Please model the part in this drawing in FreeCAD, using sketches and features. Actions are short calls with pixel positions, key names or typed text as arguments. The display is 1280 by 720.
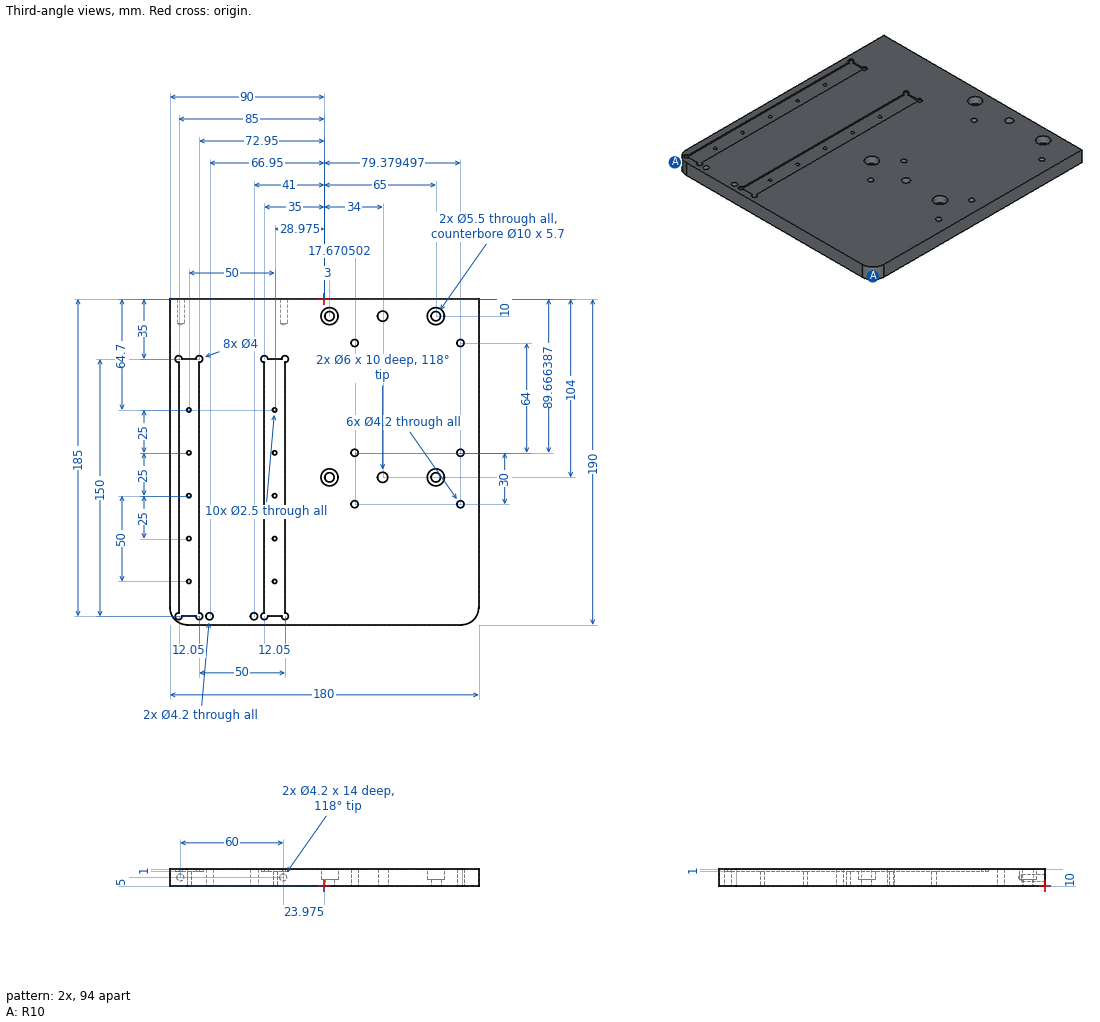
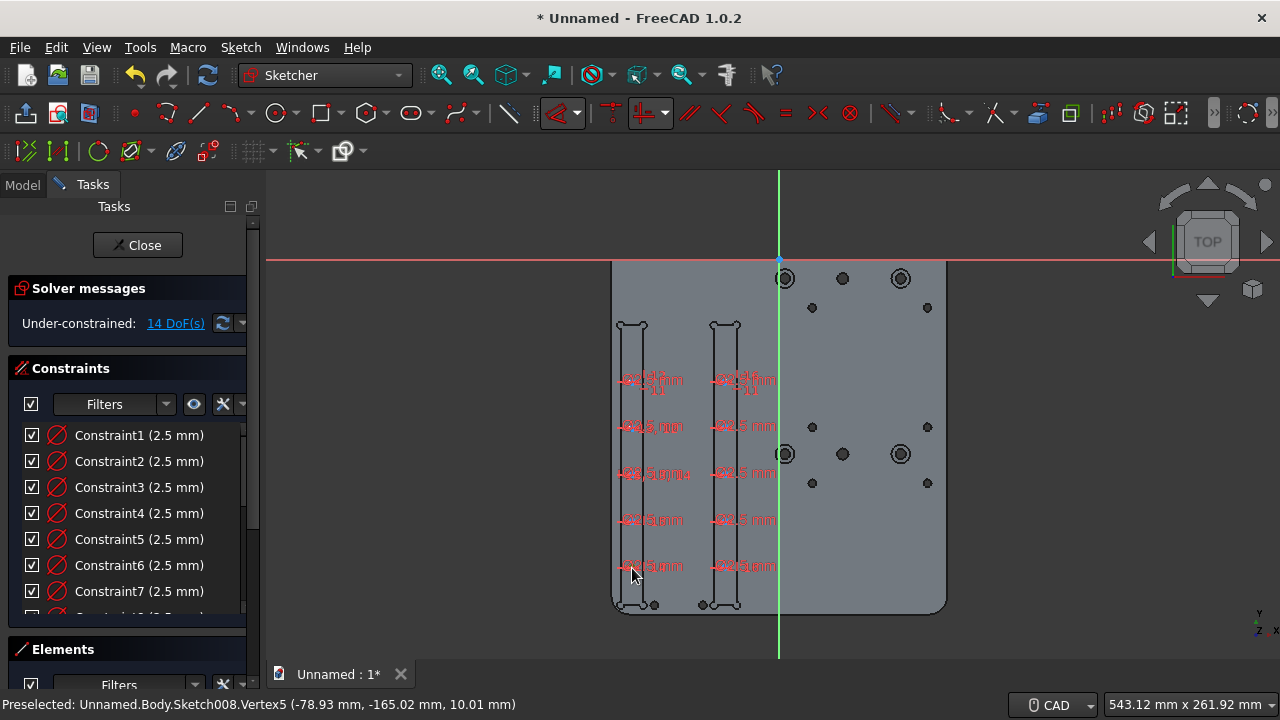
click(725, 568)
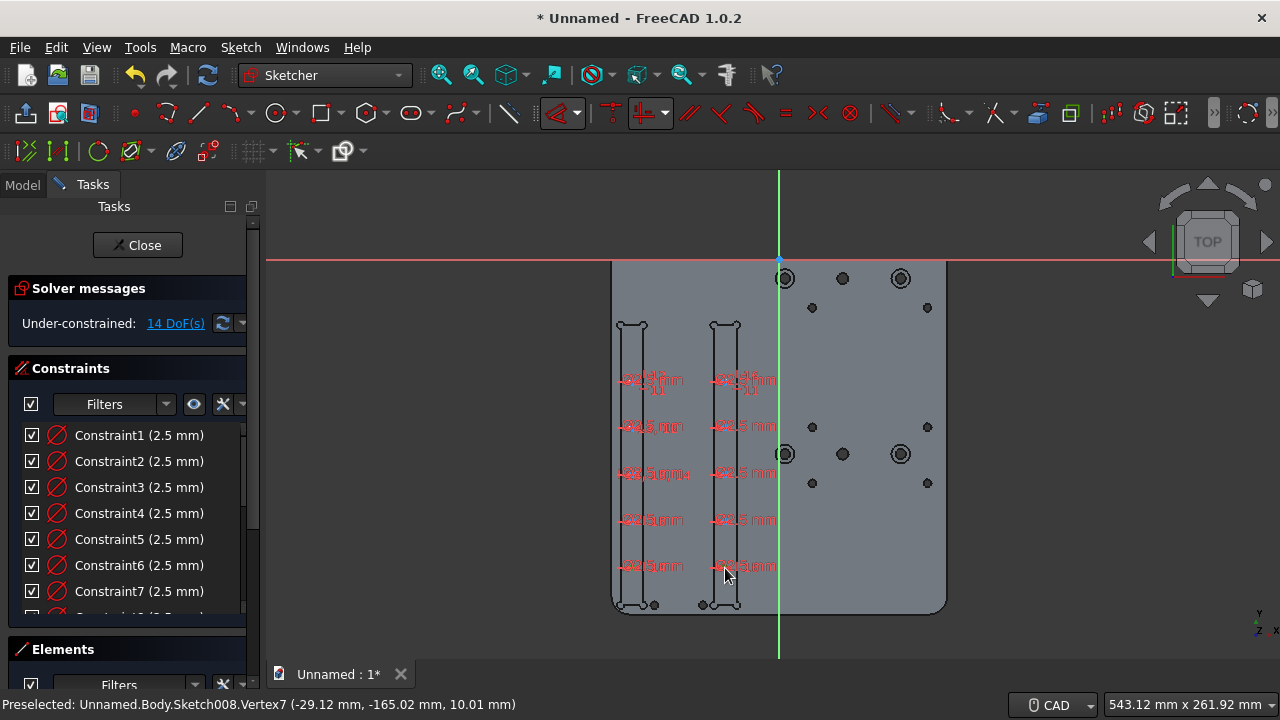
key(h)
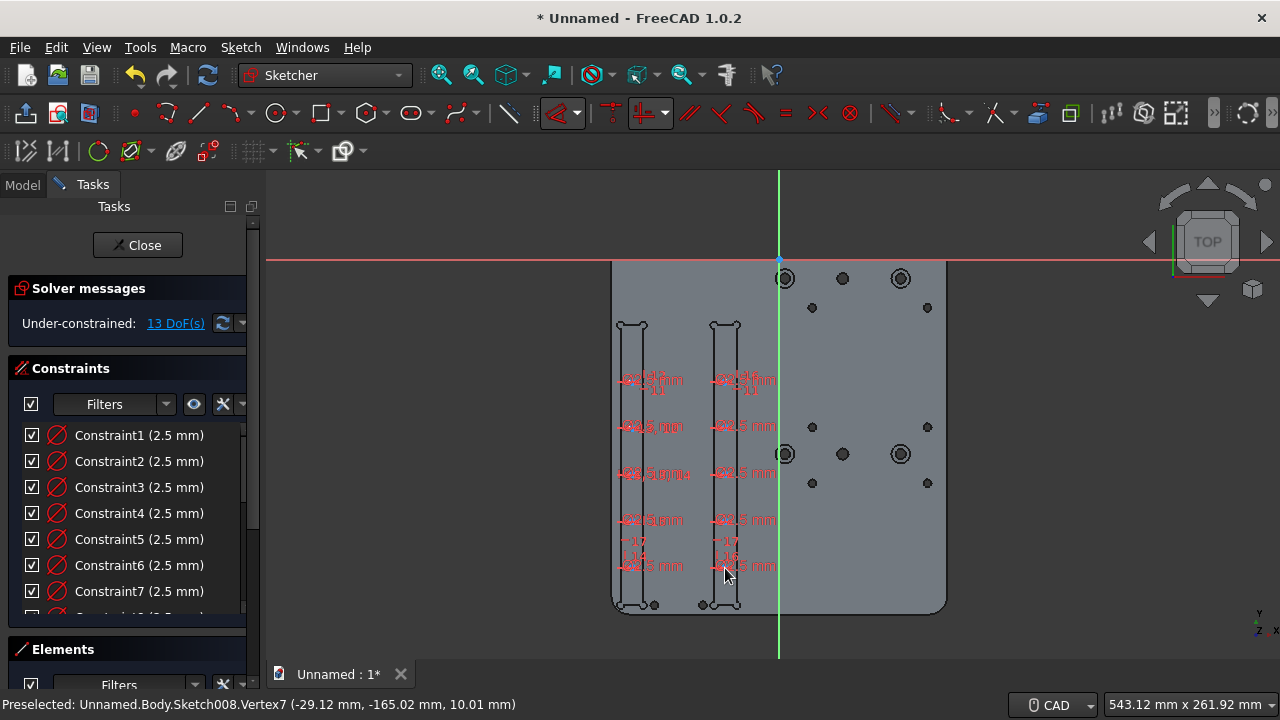
click(725, 568)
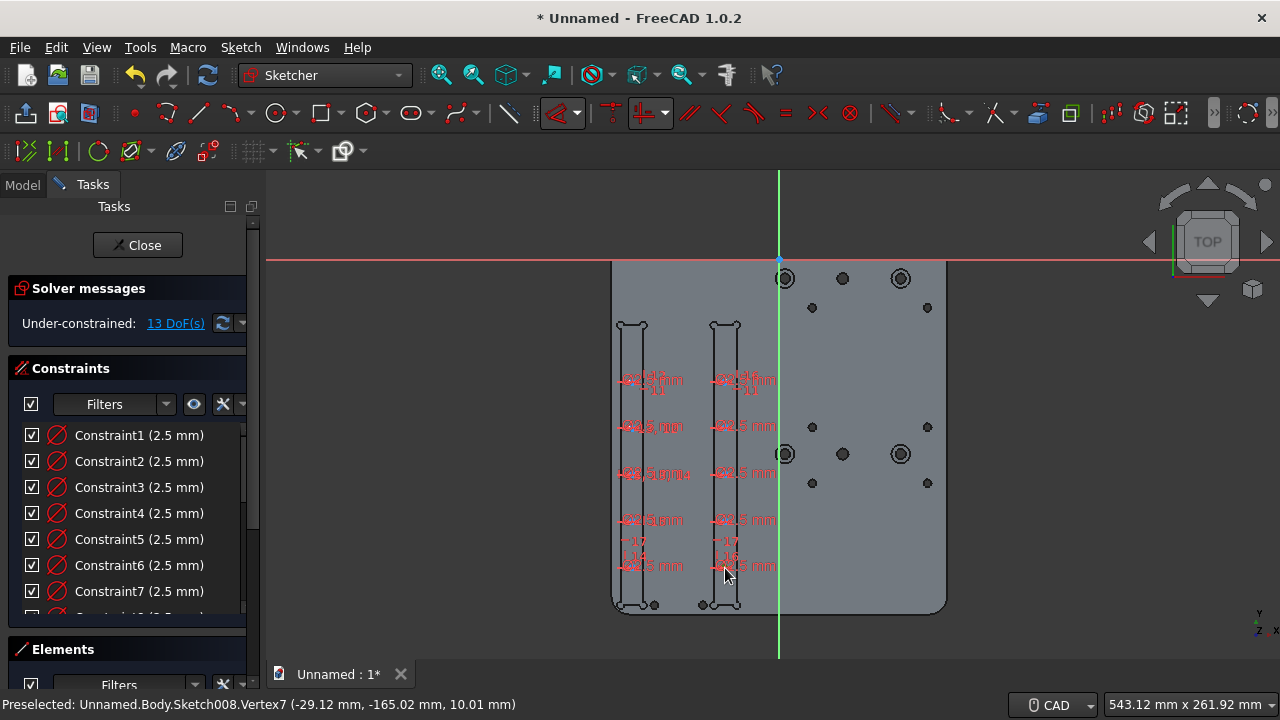
click(725, 522)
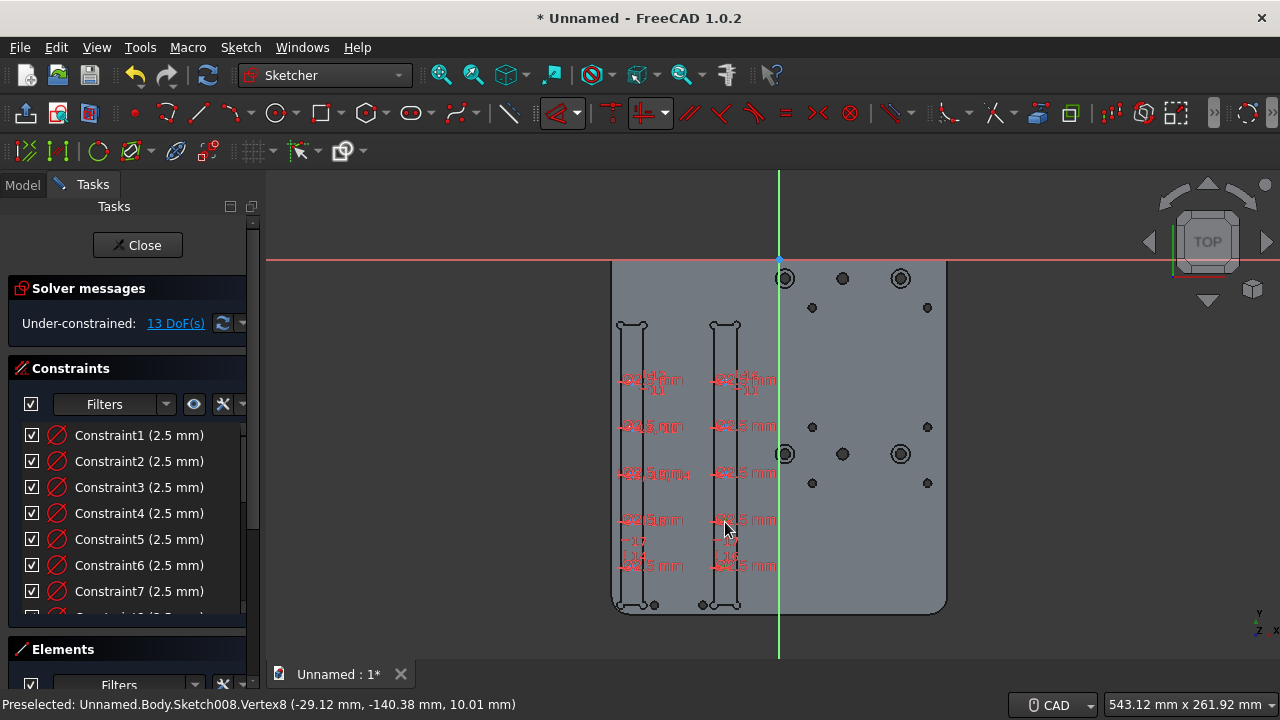
key(v)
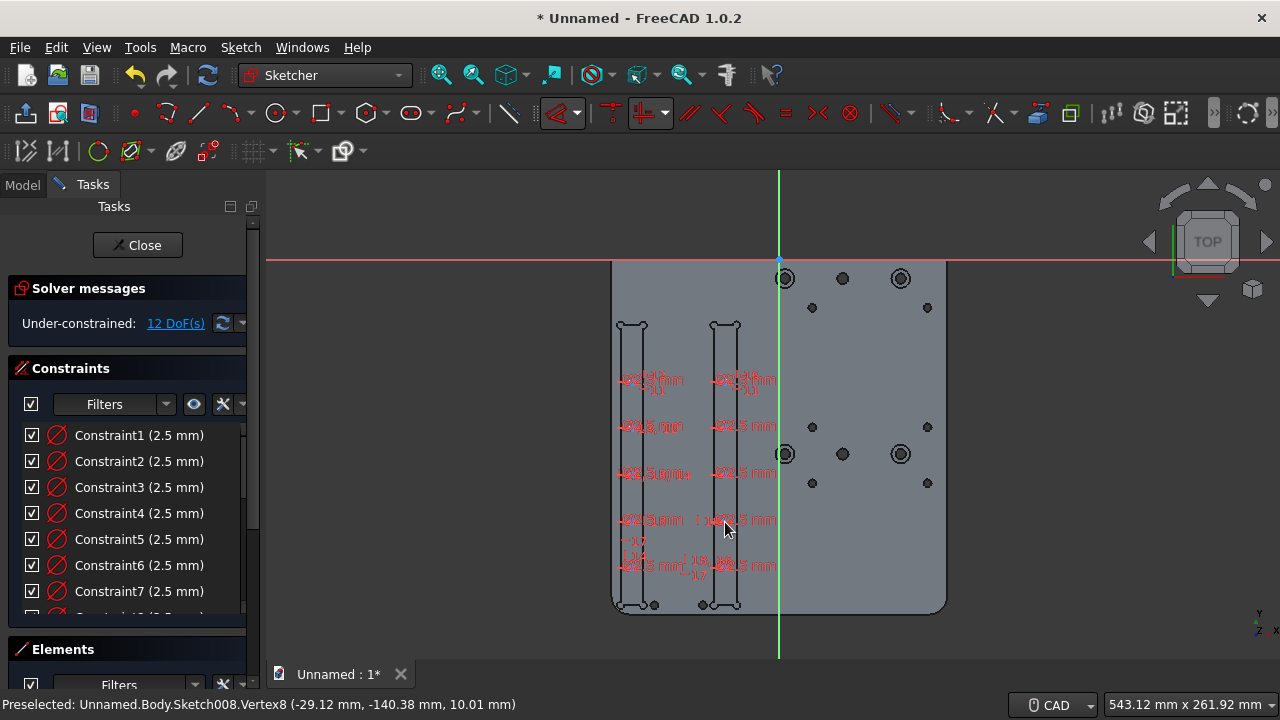
click(632, 522)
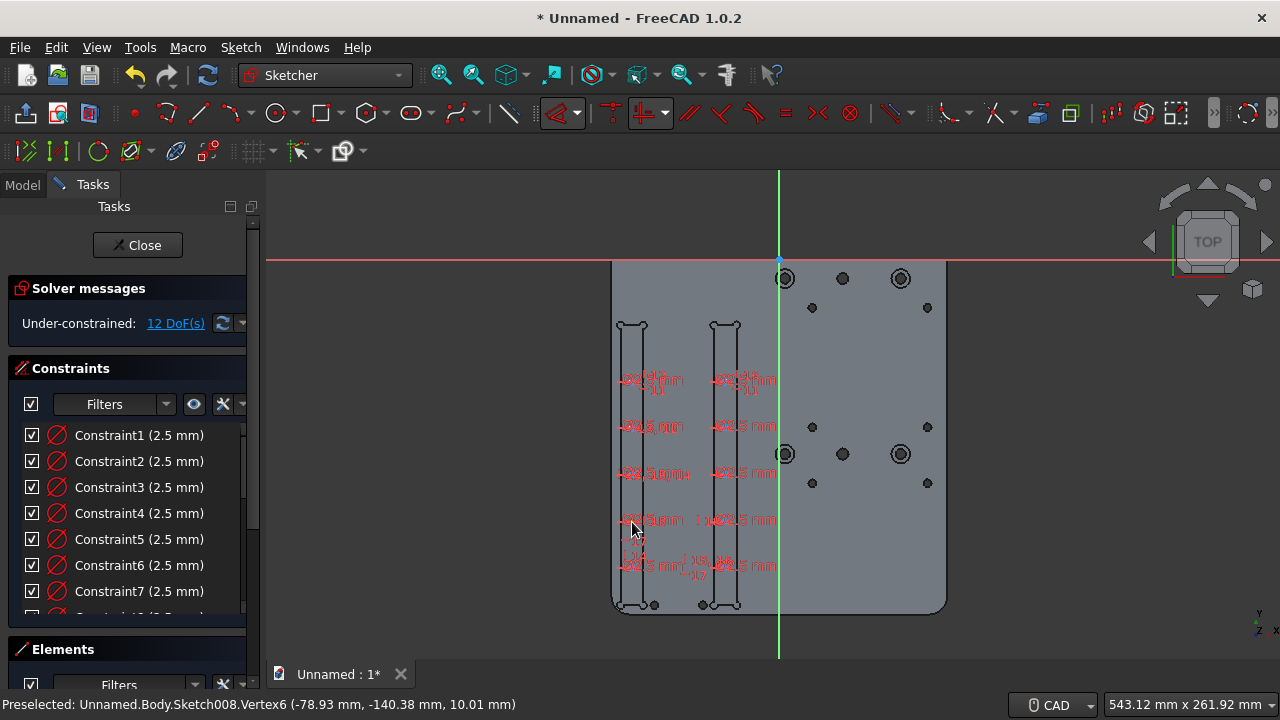
click(725, 522)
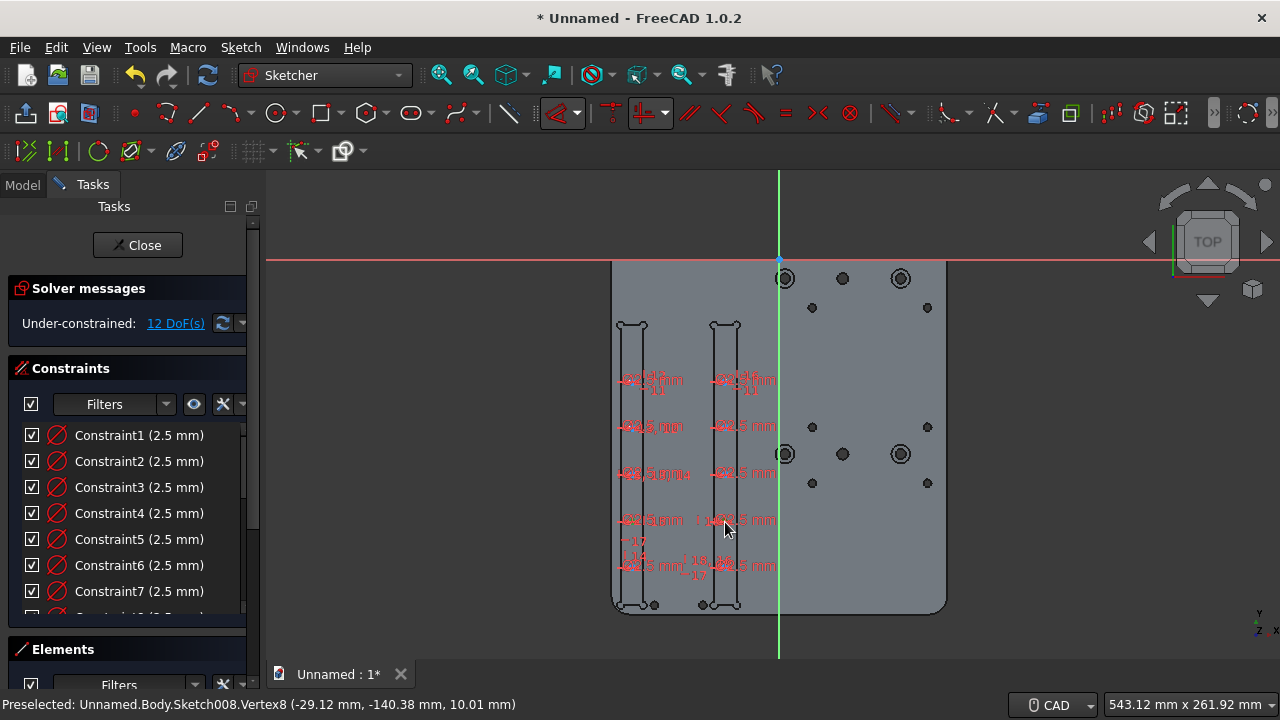
key(h)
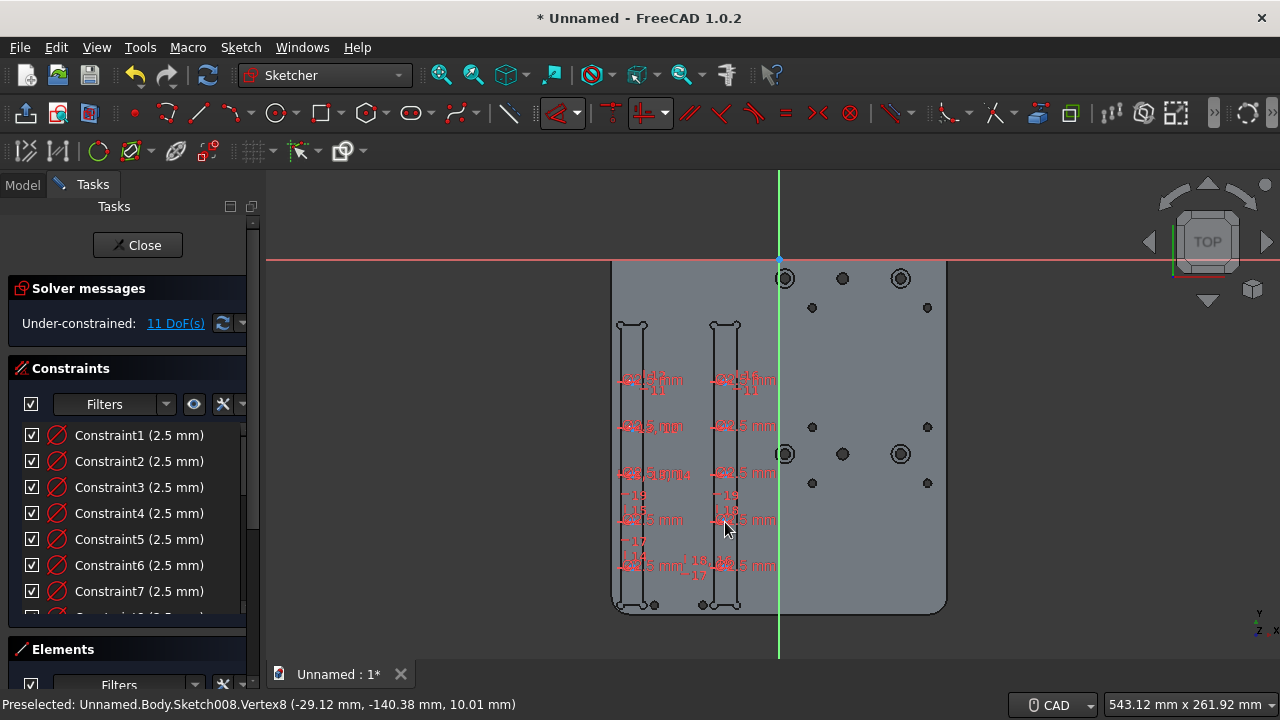
click(725, 522)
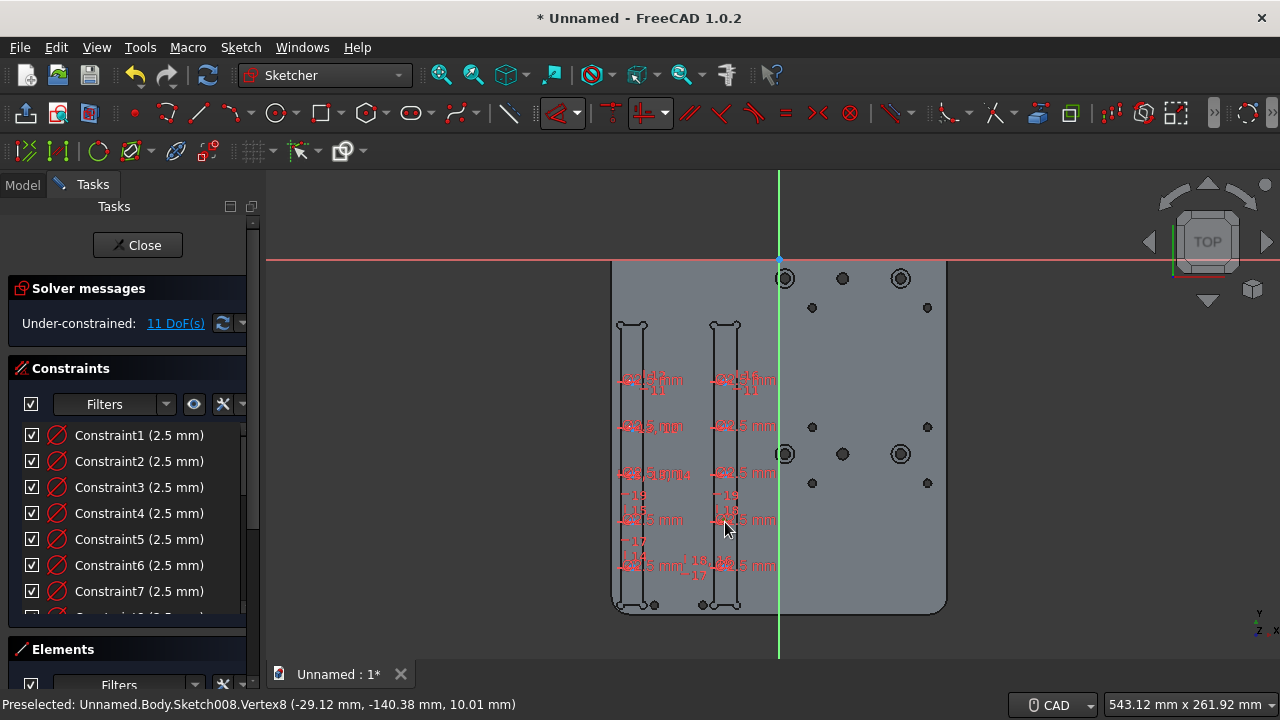
click(725, 475)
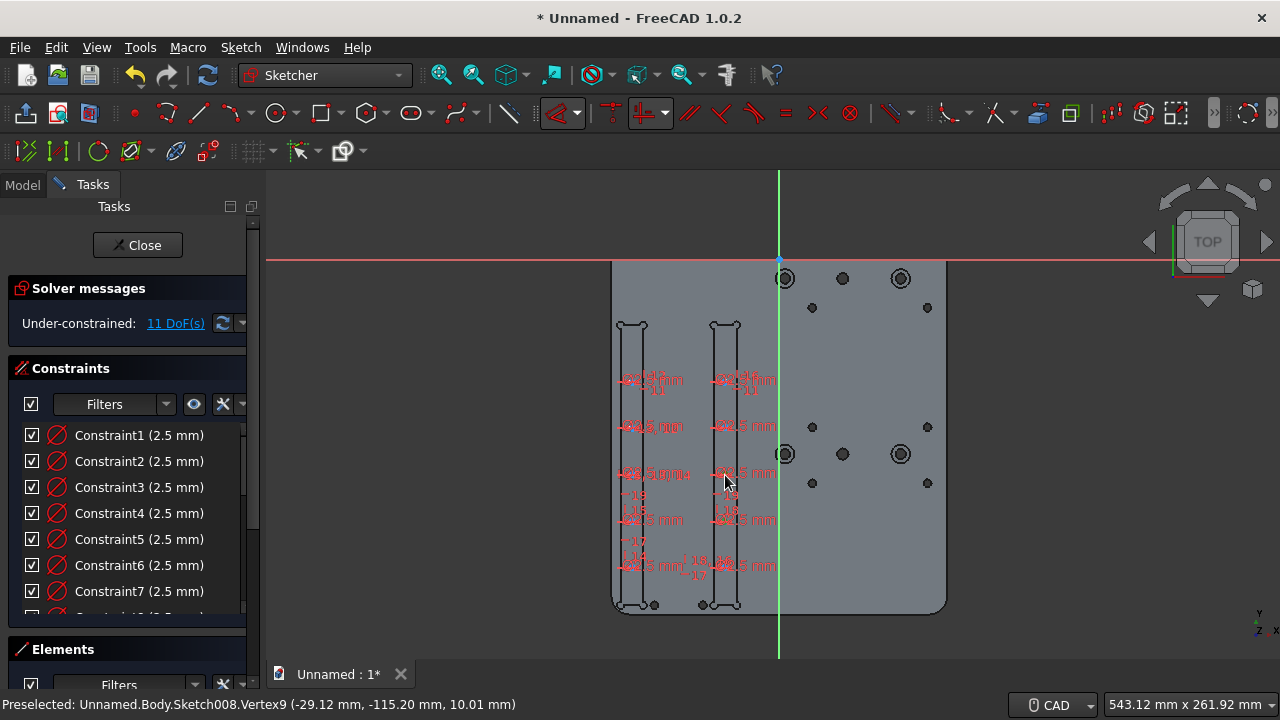
click(668, 114)